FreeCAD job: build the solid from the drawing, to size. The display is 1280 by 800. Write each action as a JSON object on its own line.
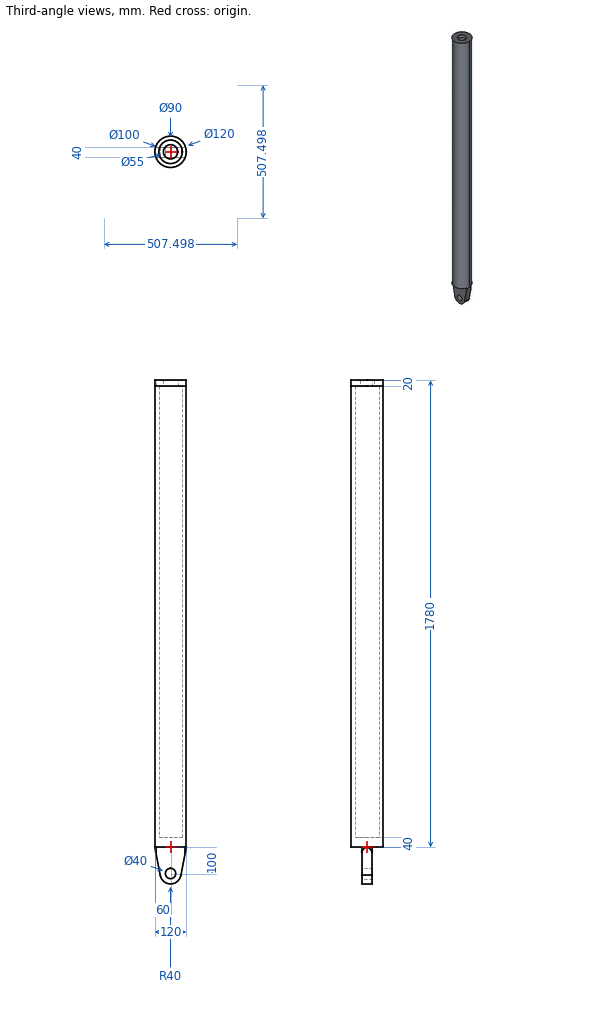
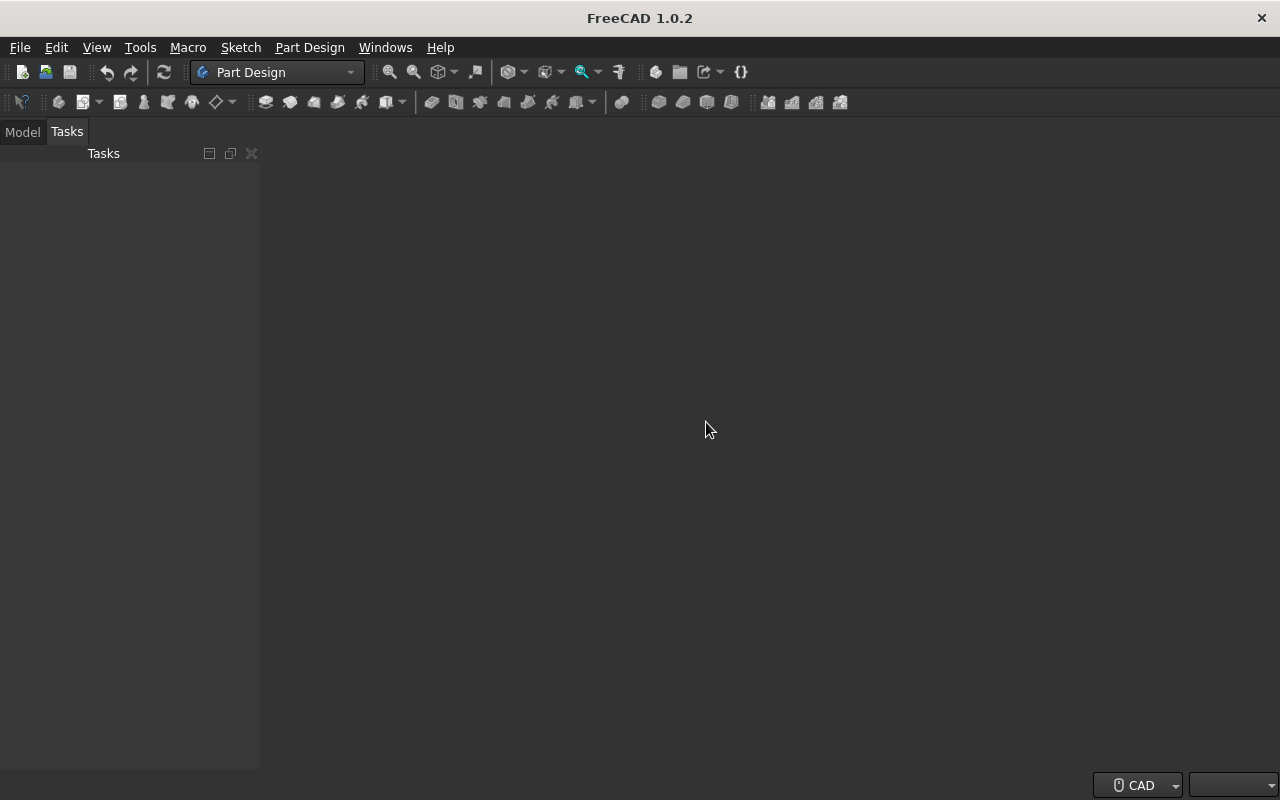
{"action": "key", "text": "ctrl+n"}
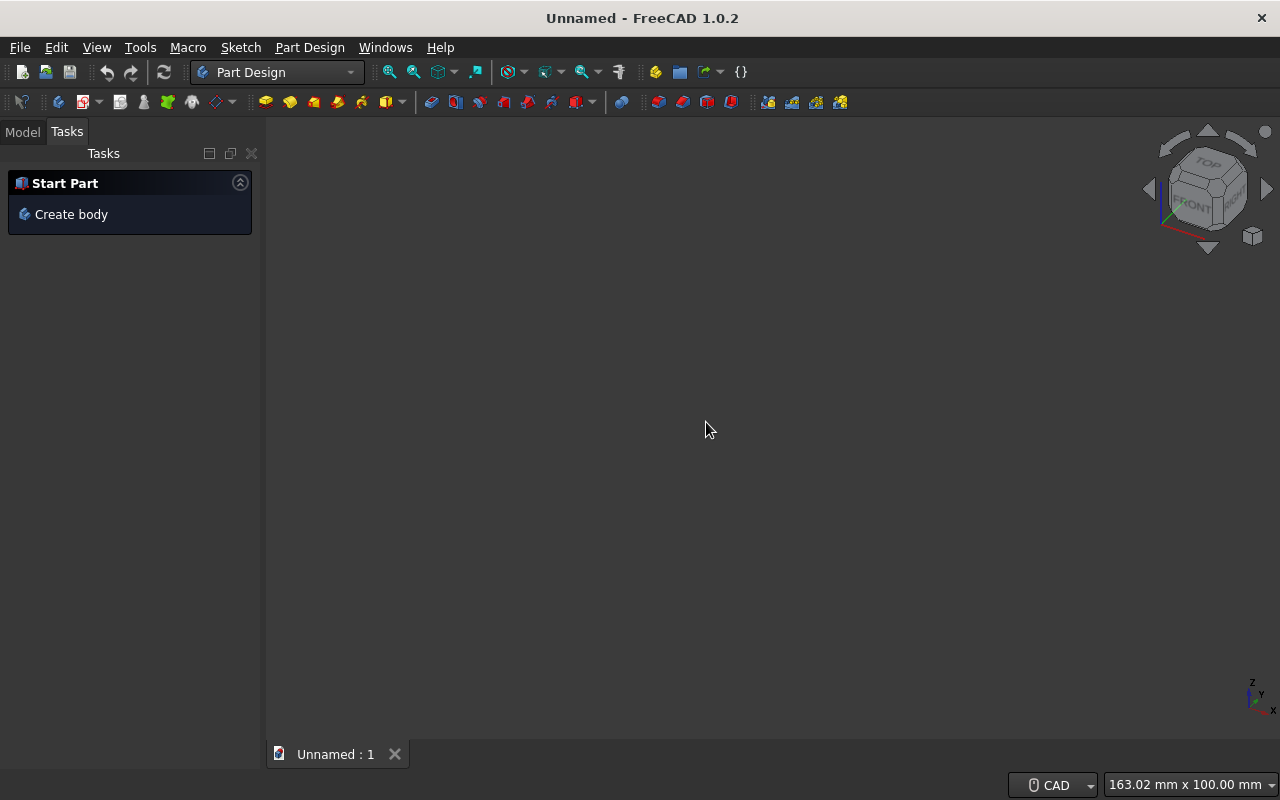
{"action": "left_click", "coordinate": [84, 102]}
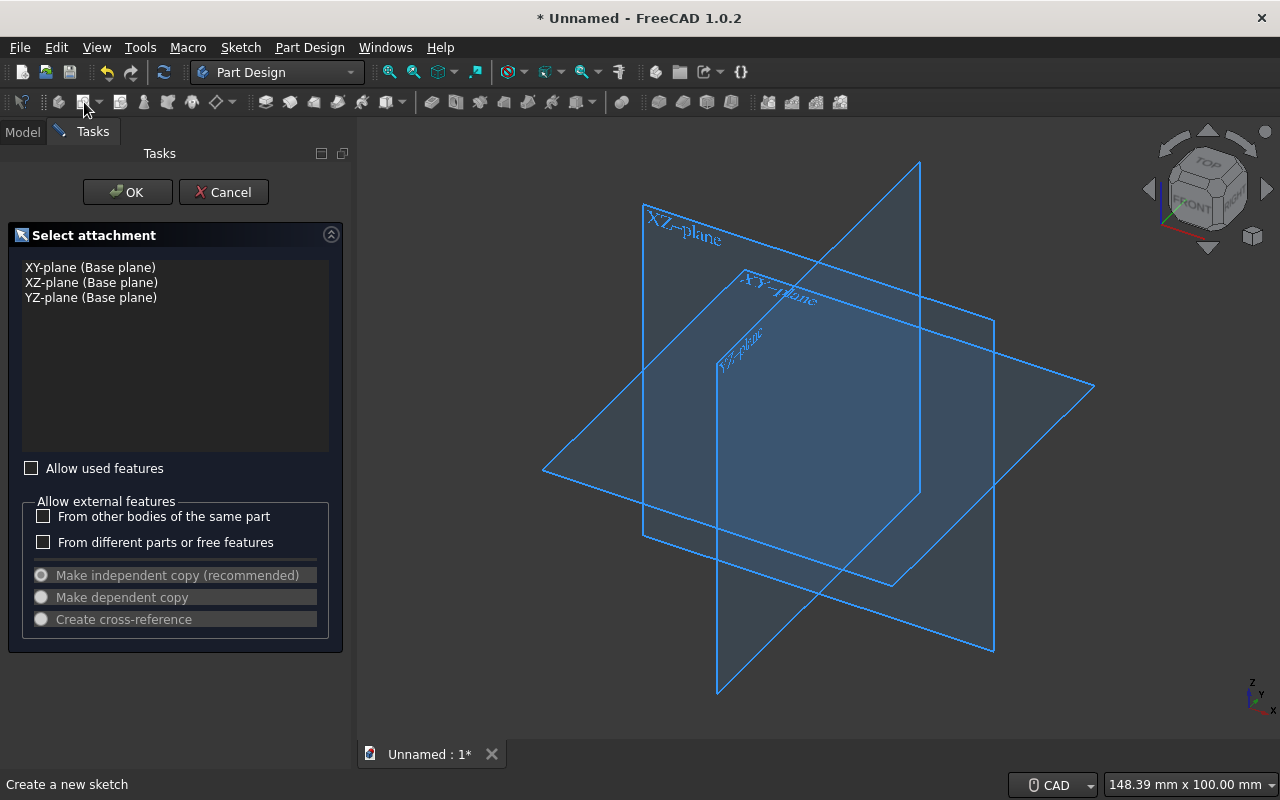
{"action": "left_click", "coordinate": [82, 268]}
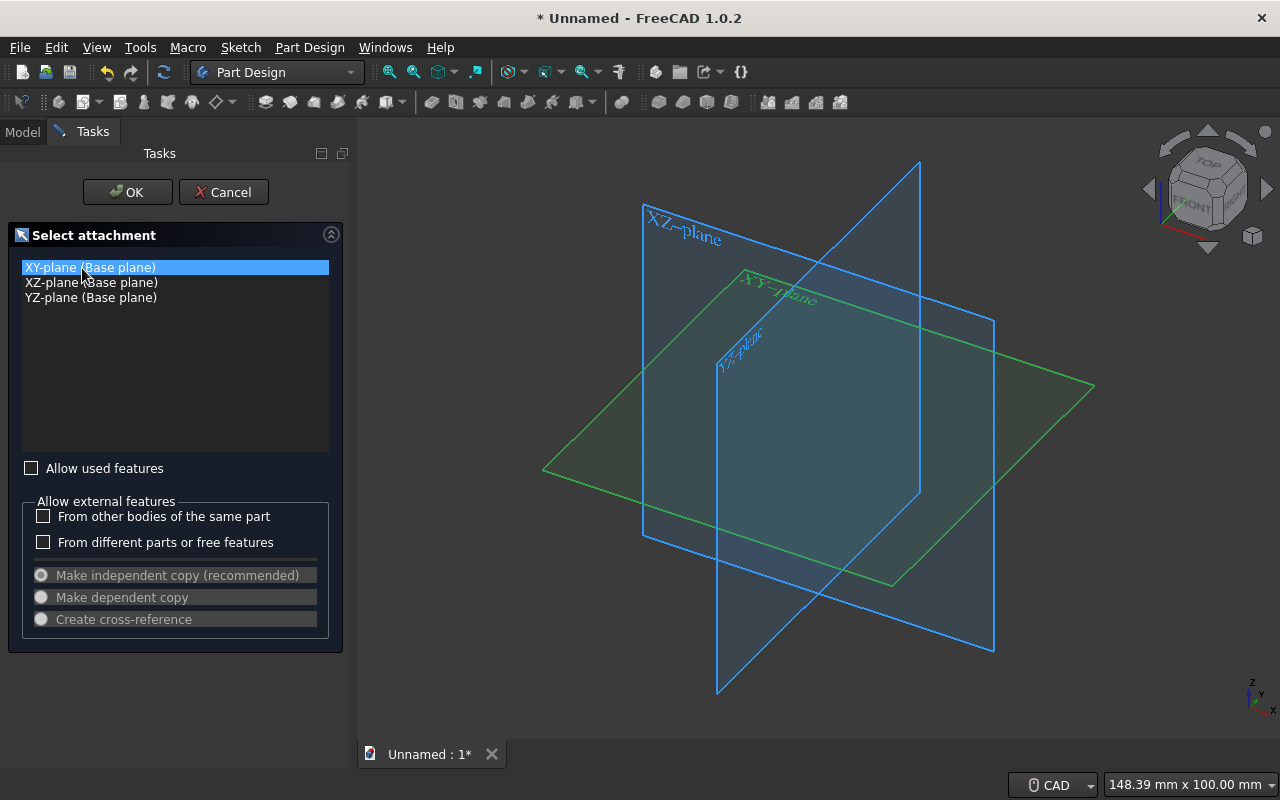
{"action": "left_click", "coordinate": [128, 192]}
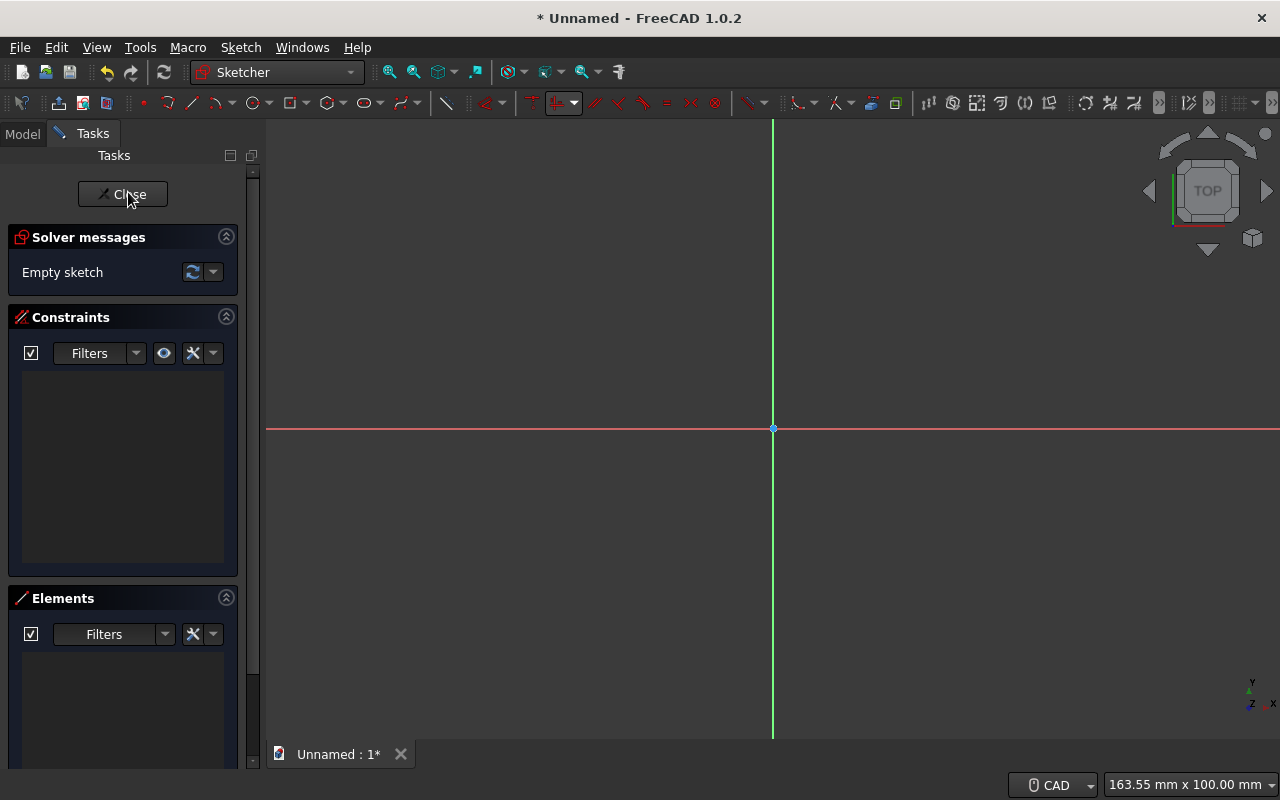
{"action": "scroll", "coordinate": [621, 429], "scroll_direction": "down", "scroll_amount": 3}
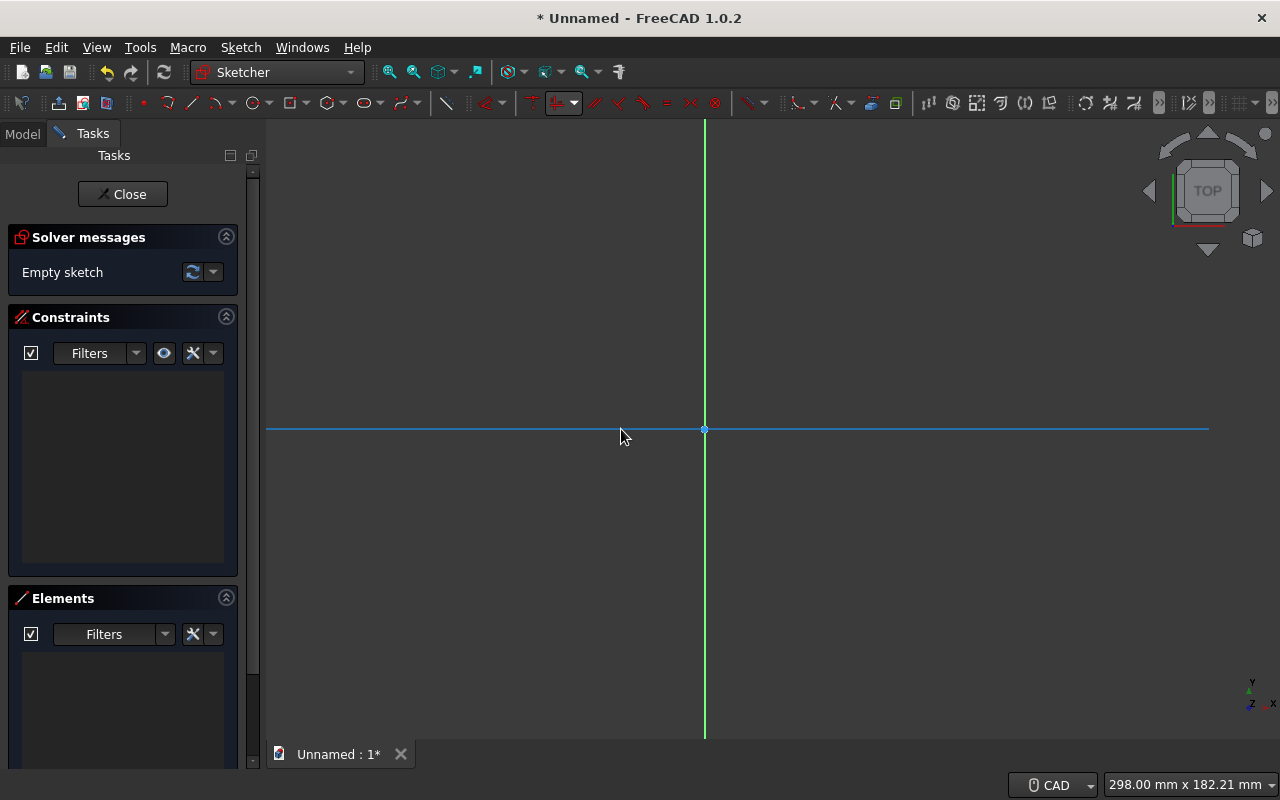
{"action": "left_click", "coordinate": [254, 104]}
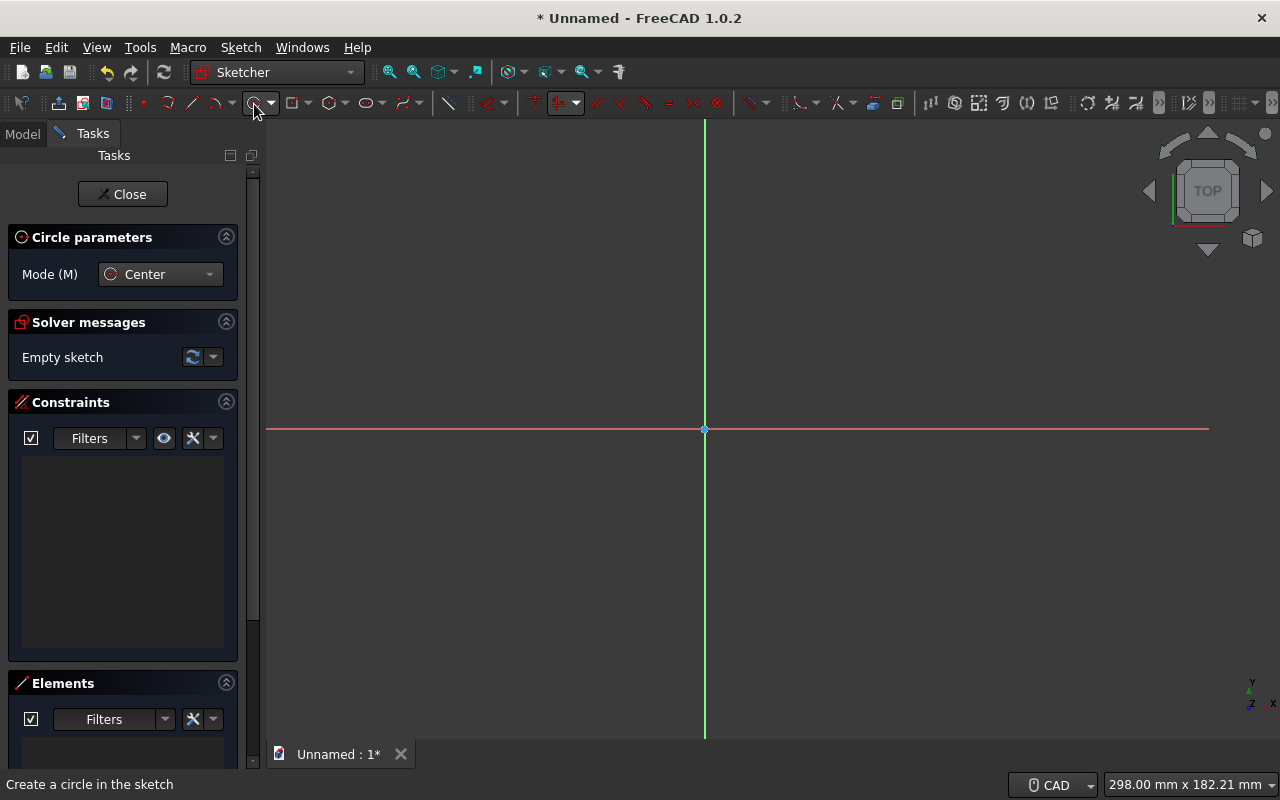
{"action": "left_click", "coordinate": [705, 429]}
{"action": "mouse_move", "coordinate": [849, 285]}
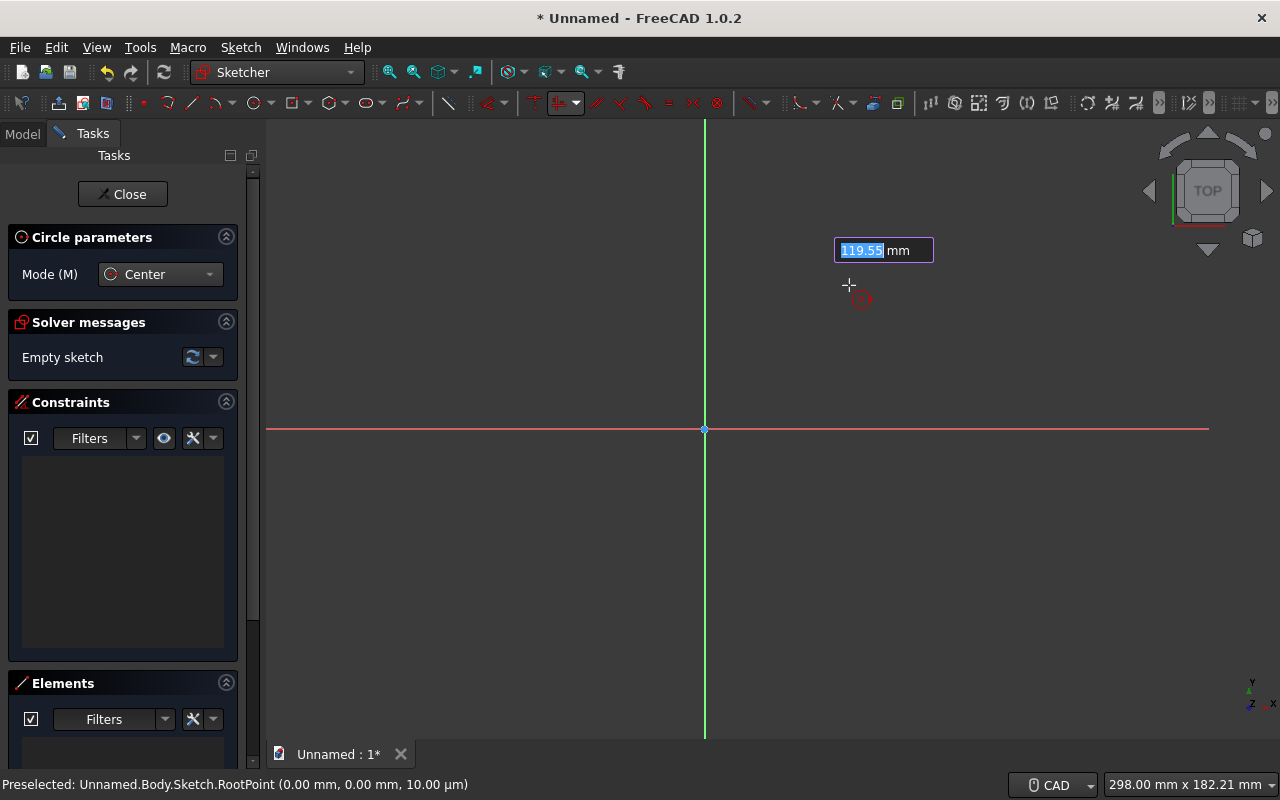
{"action": "type", "text": "120"}
{"action": "key", "text": "Return"}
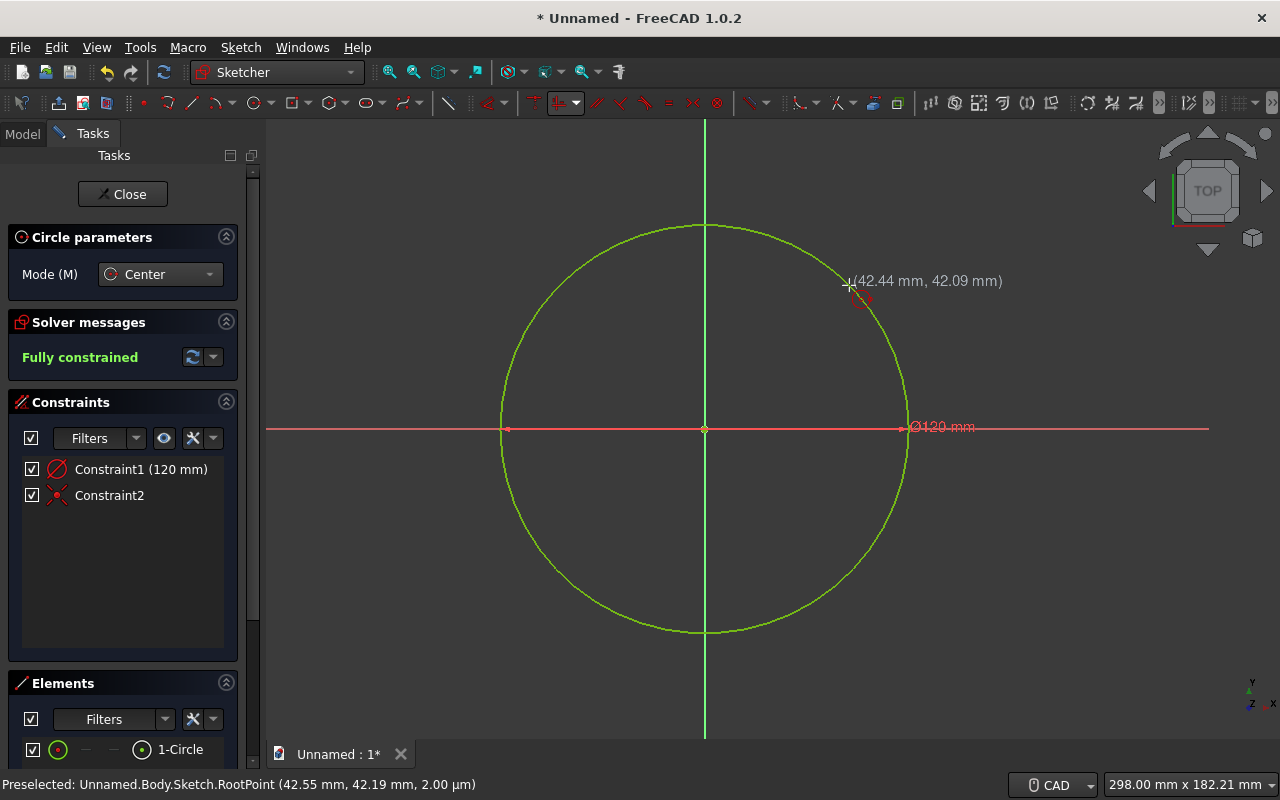
{"action": "left_click", "coordinate": [705, 429]}
{"action": "mouse_move", "coordinate": [813, 321]}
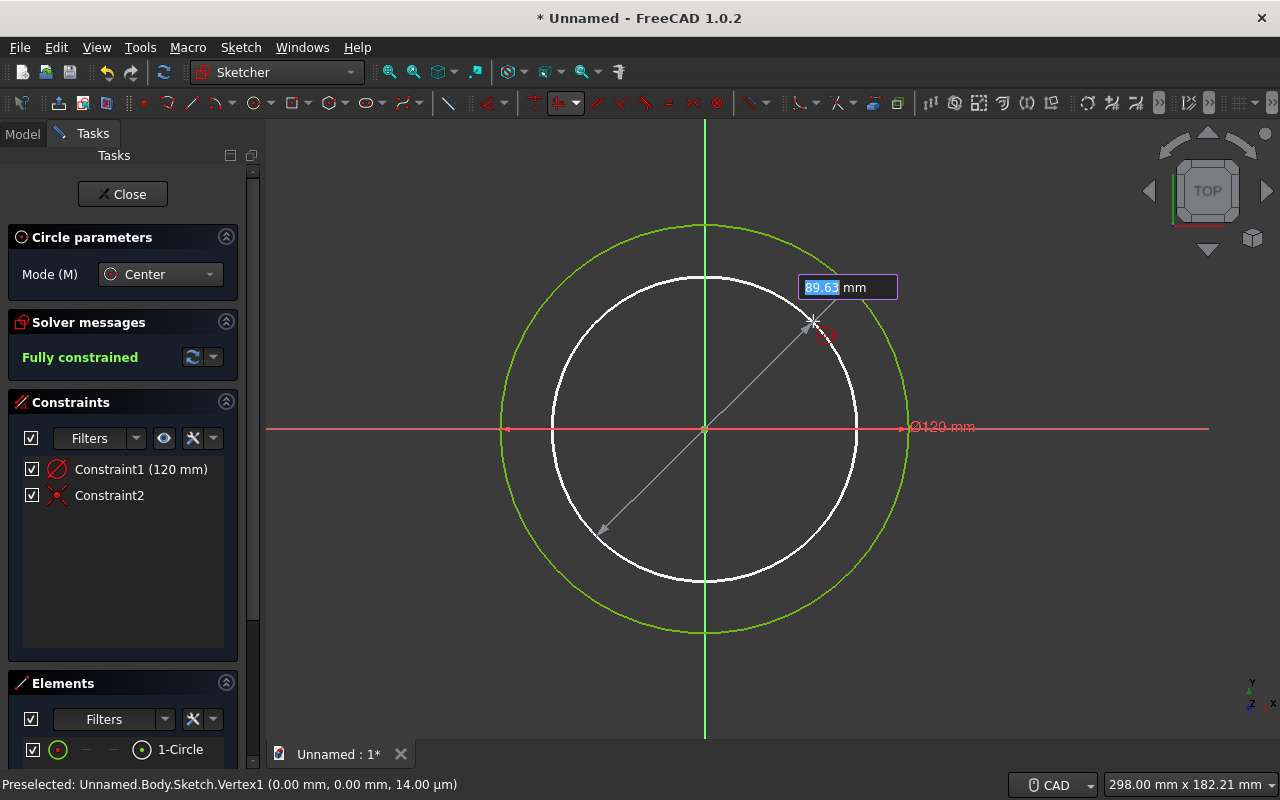
{"action": "type", "text": "90"}
{"action": "key", "text": "Return"}
{"action": "key", "text": "Escape"}